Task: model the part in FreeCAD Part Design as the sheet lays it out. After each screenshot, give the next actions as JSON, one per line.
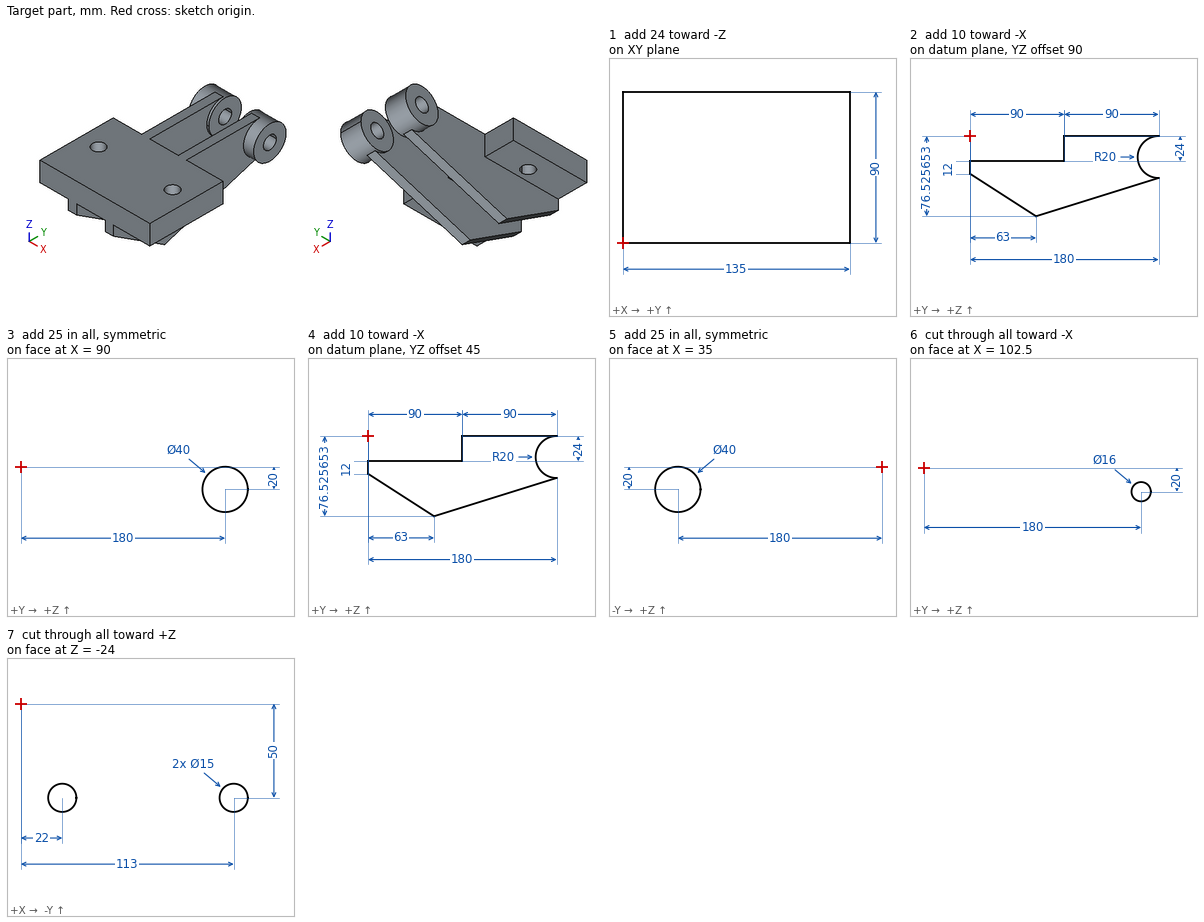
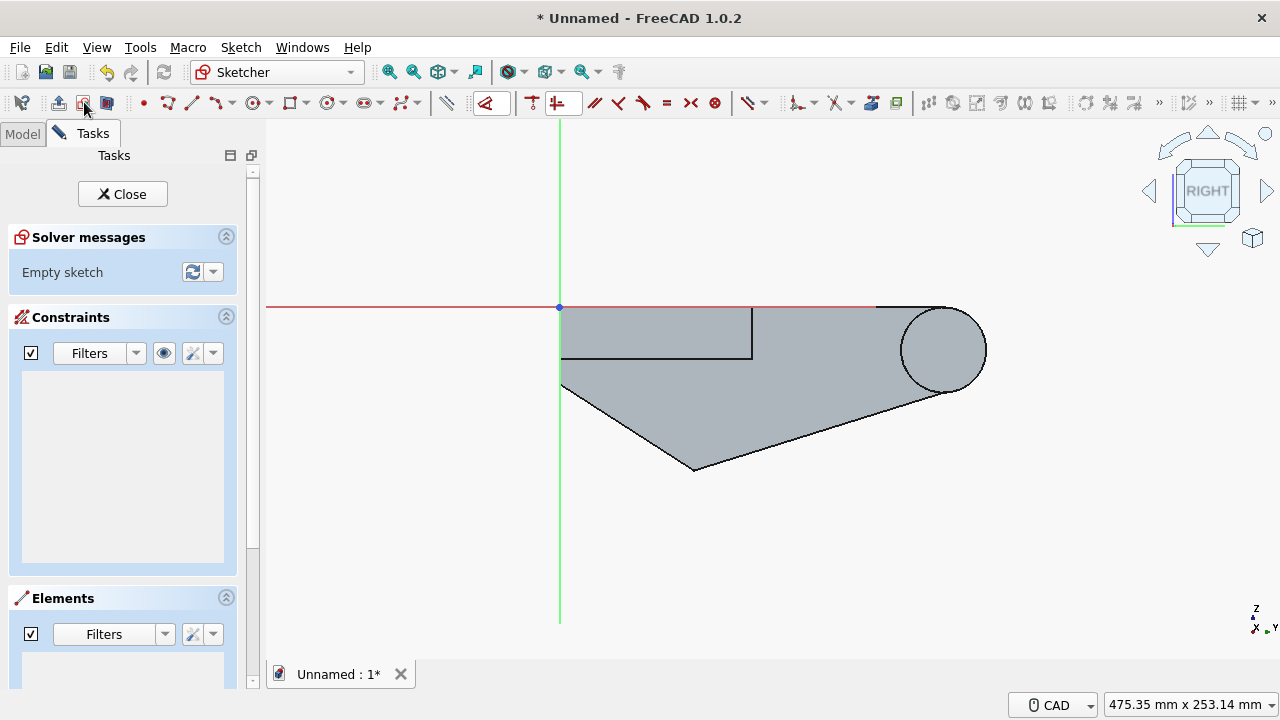
{"action": "scroll", "coordinate": [968, 346], "scroll_direction": "up", "scroll_amount": 12}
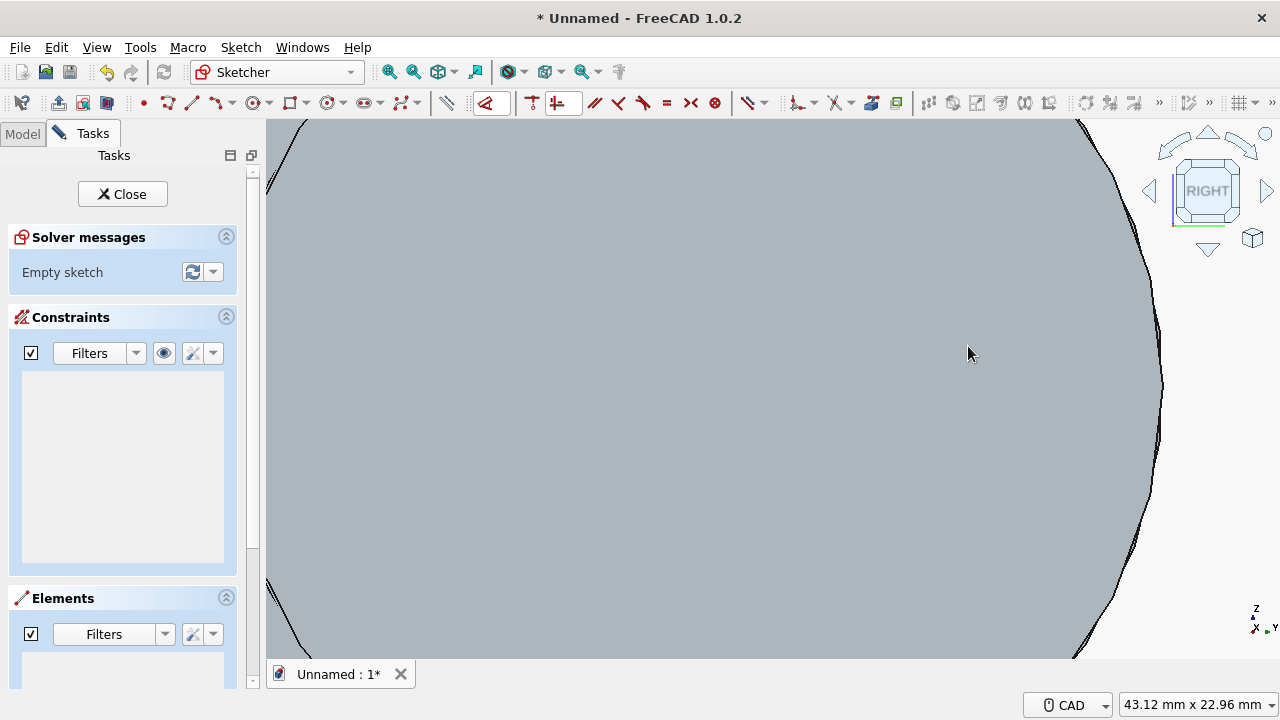
{"action": "left_click", "coordinate": [254, 104]}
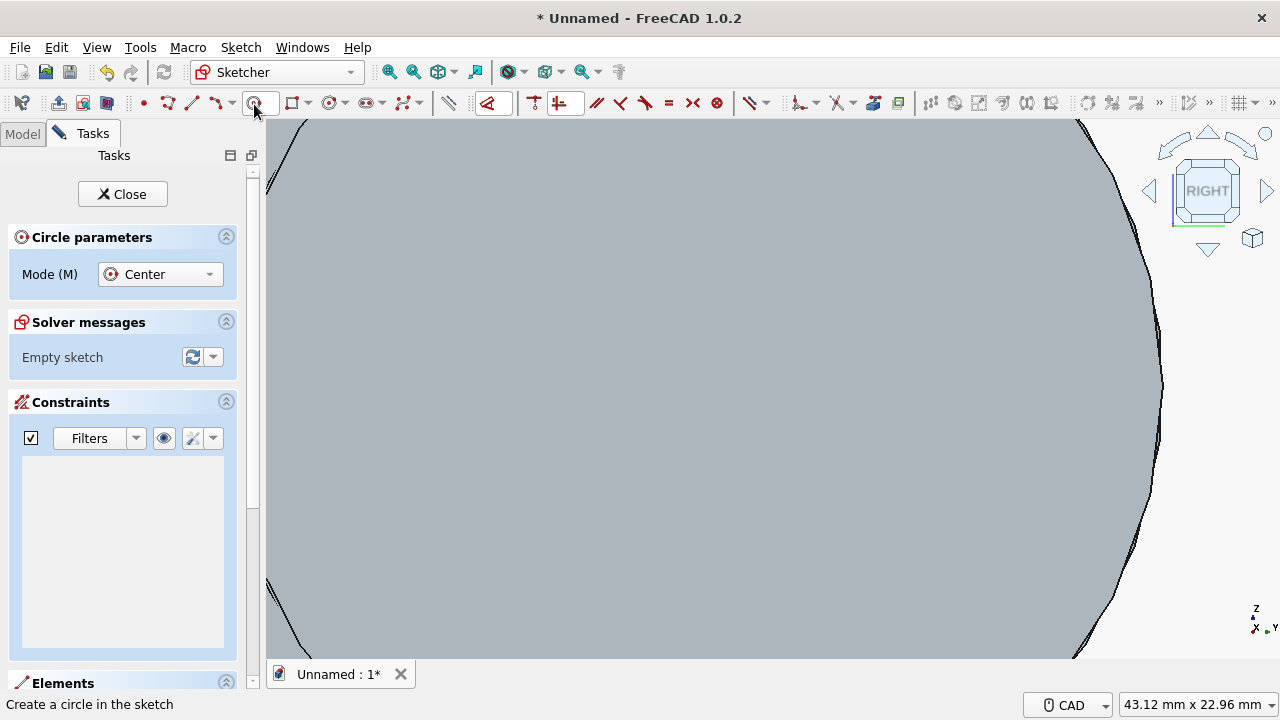
{"action": "left_click", "coordinate": [693, 386]}
{"action": "mouse_move", "coordinate": [826, 253]}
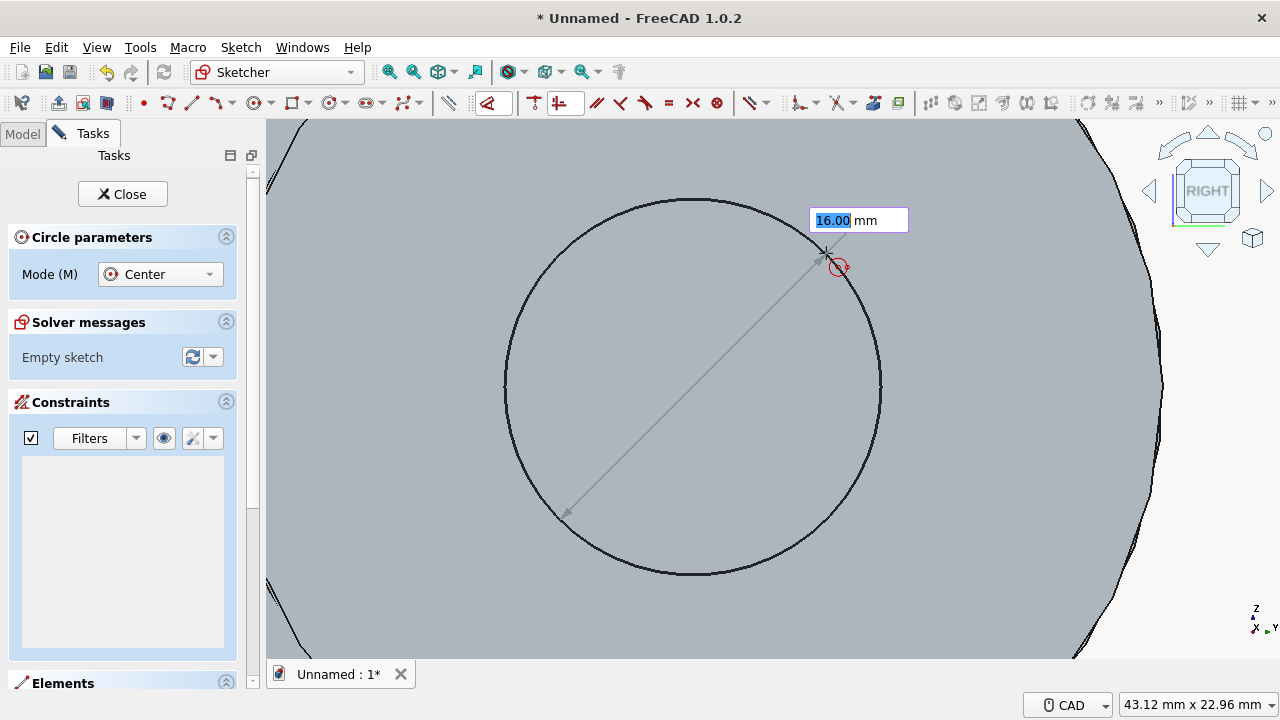
{"action": "type", "text": "16"}
{"action": "key", "text": "Return"}
{"action": "key", "text": "Escape"}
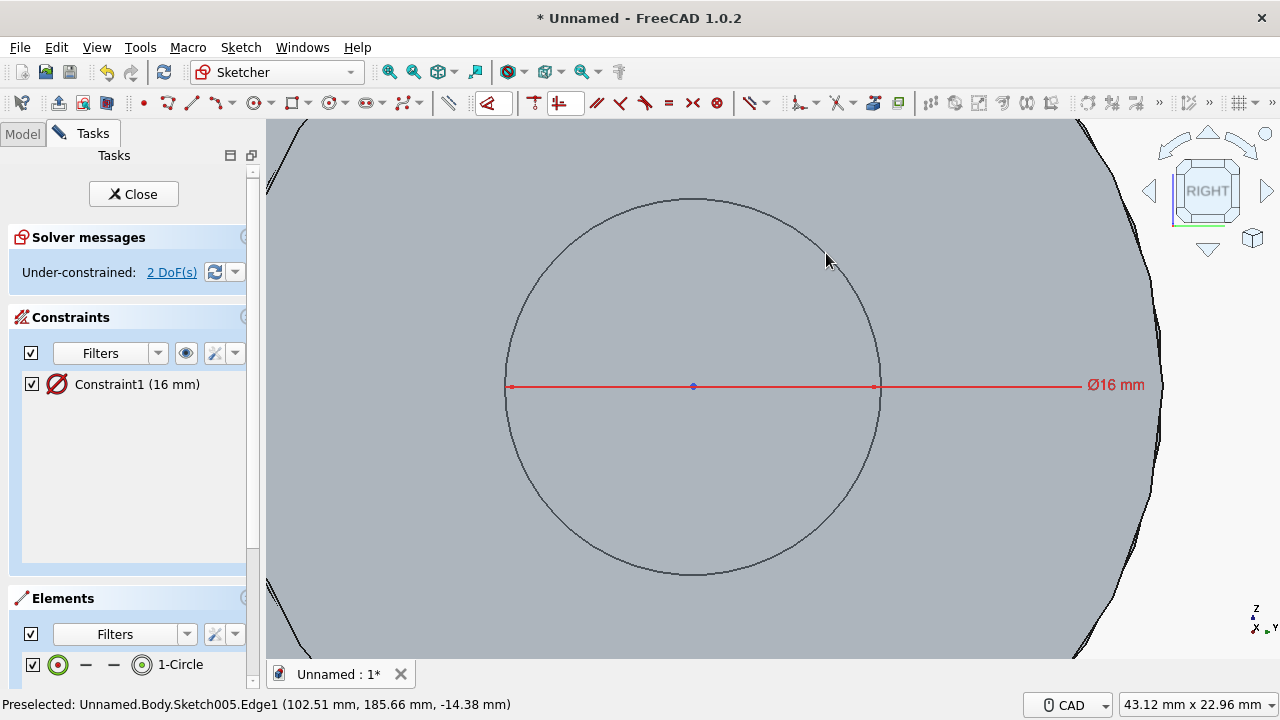
{"action": "left_click", "coordinate": [693, 387]}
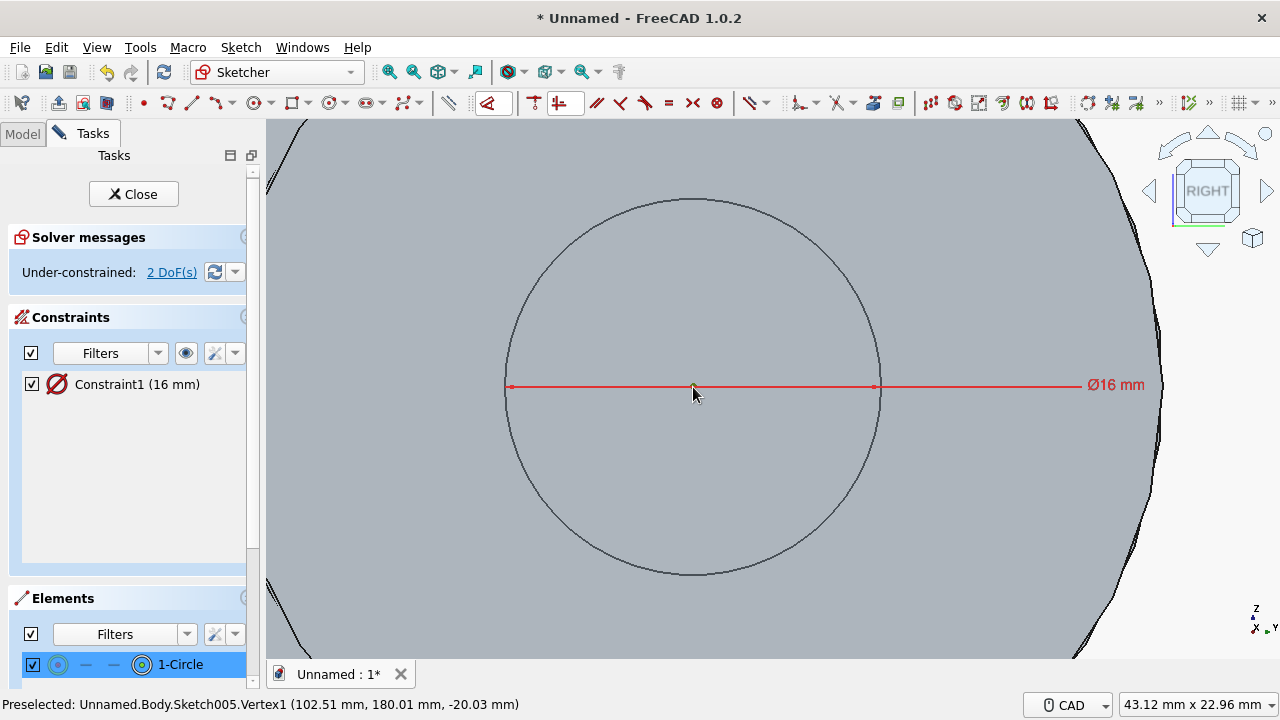
{"action": "key", "text": "i"}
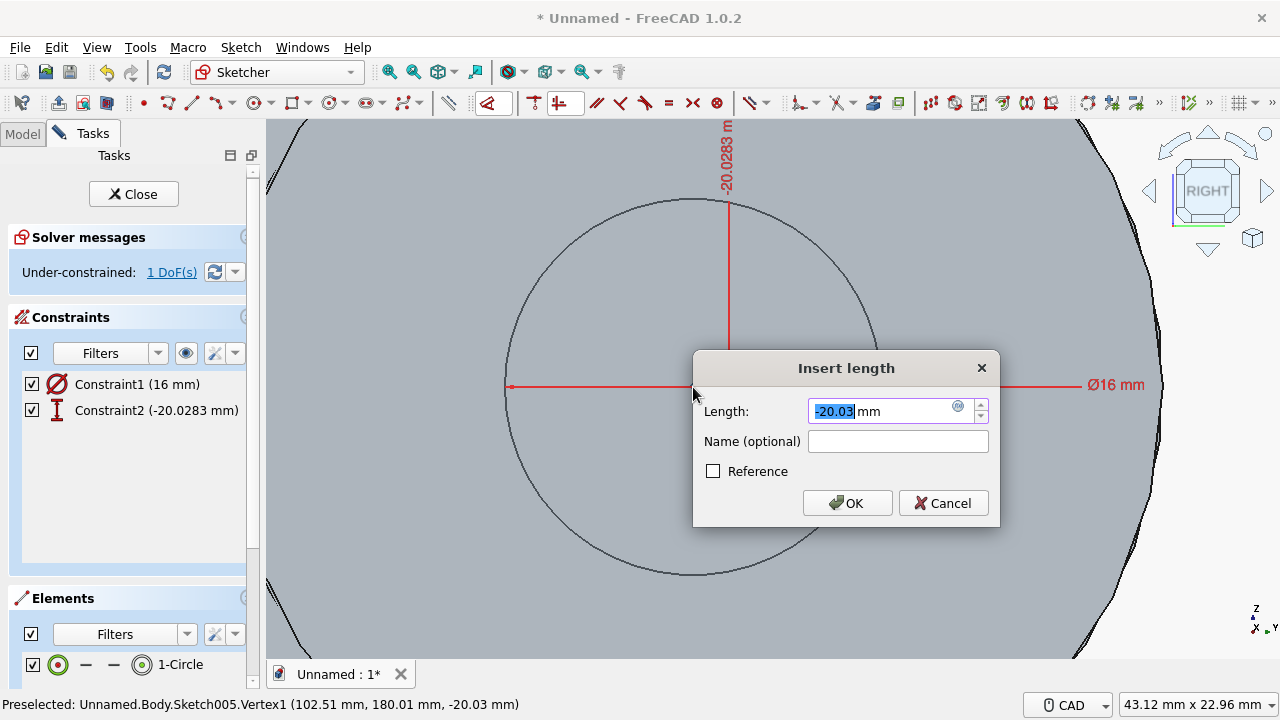
{"action": "type", "text": "-20"}
{"action": "key", "text": "Return"}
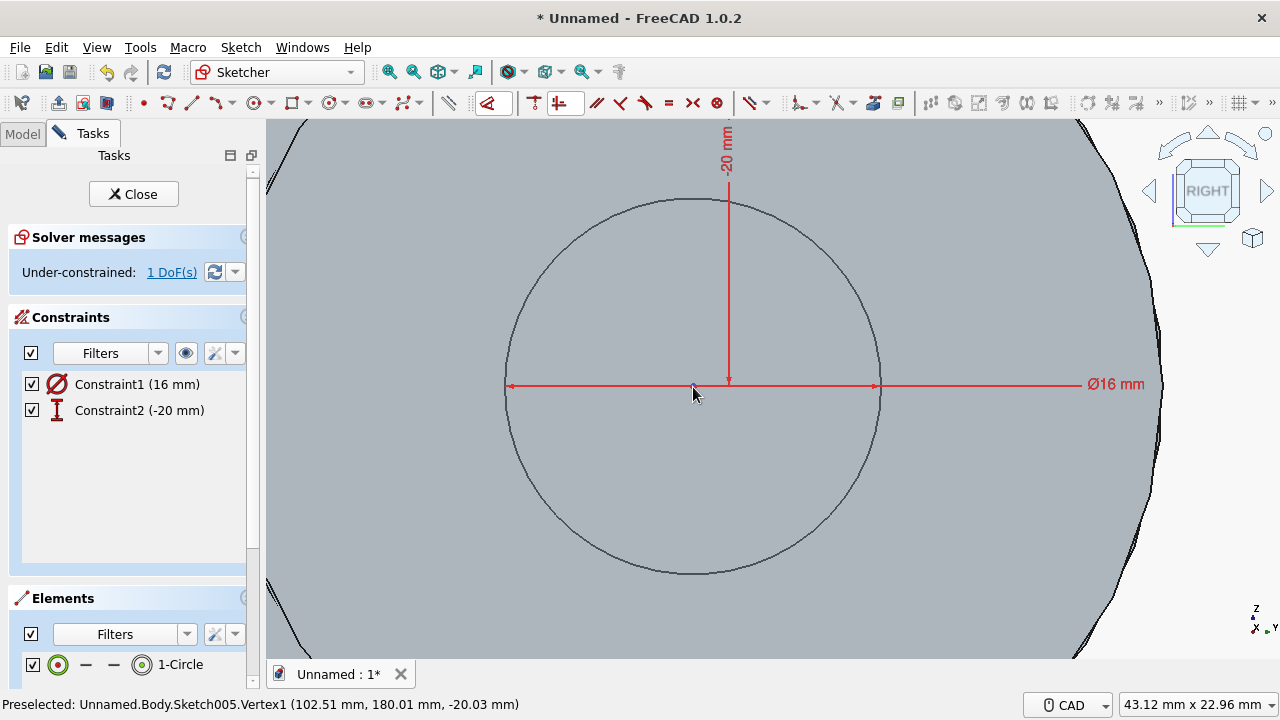
{"action": "left_click", "coordinate": [693, 386]}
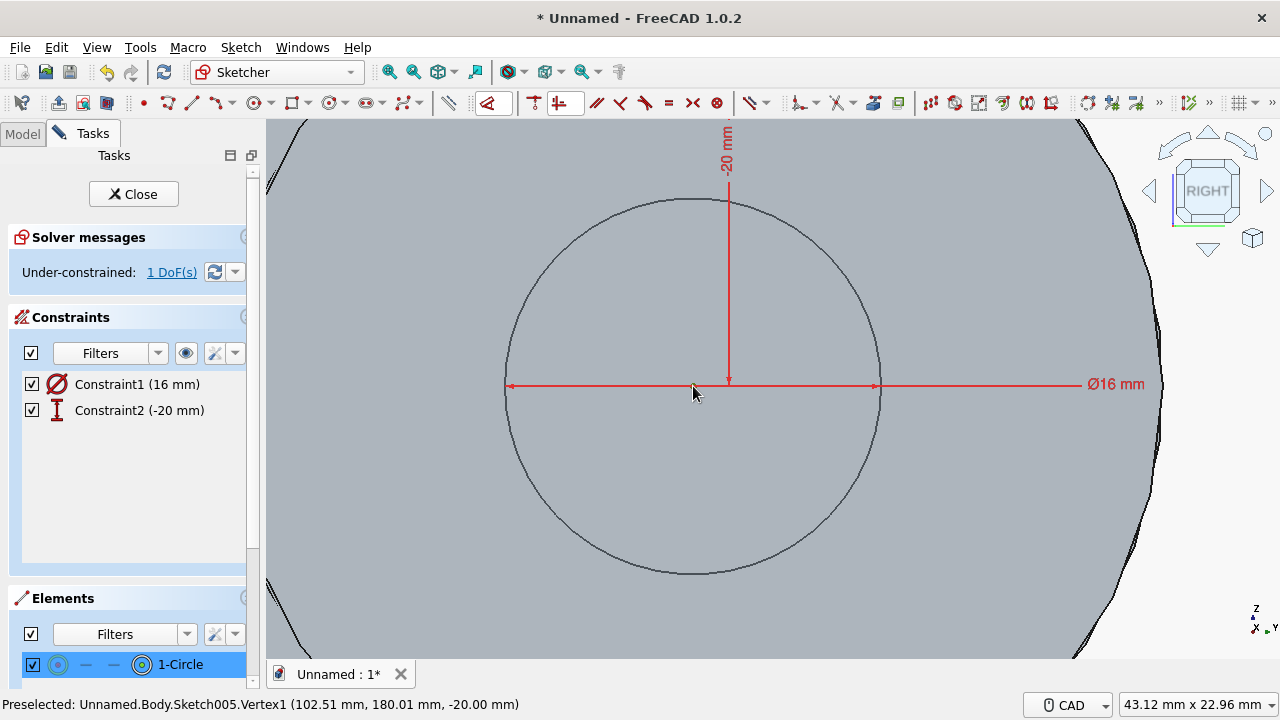
{"action": "key", "text": "l"}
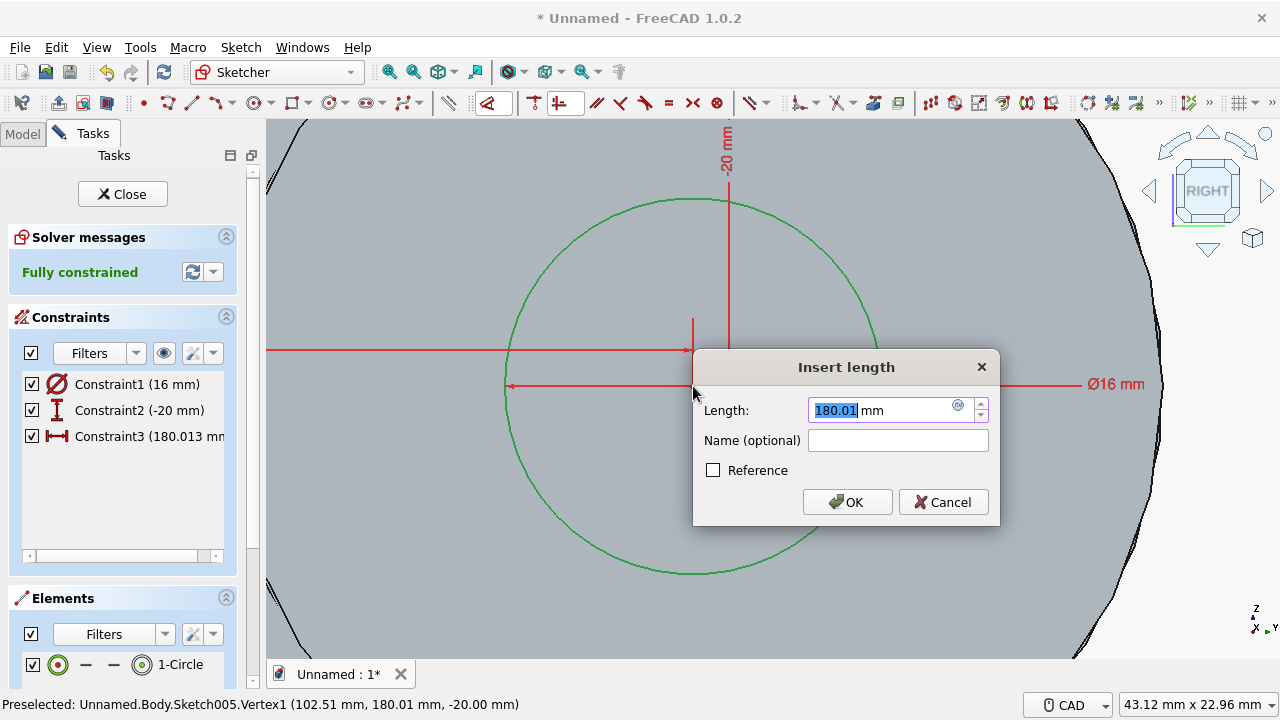
{"action": "type", "text": "180"}
{"action": "key", "text": "Return"}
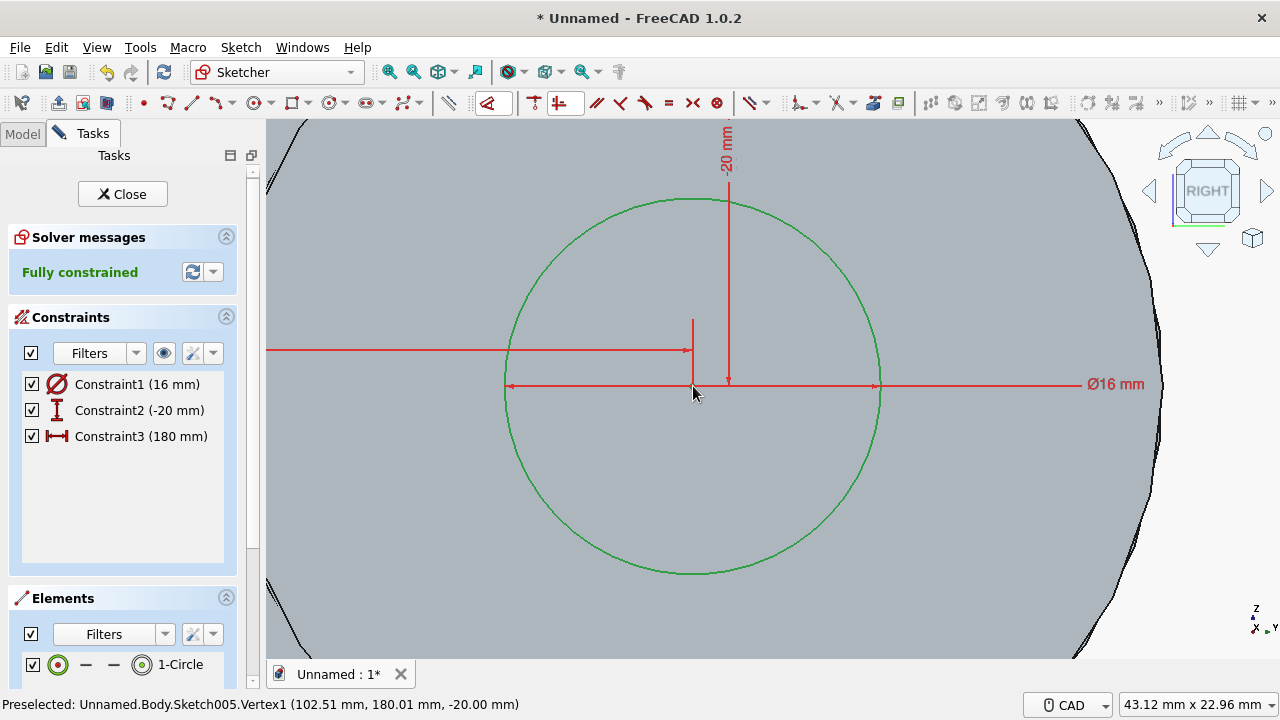
{"action": "left_click", "coordinate": [123, 194]}